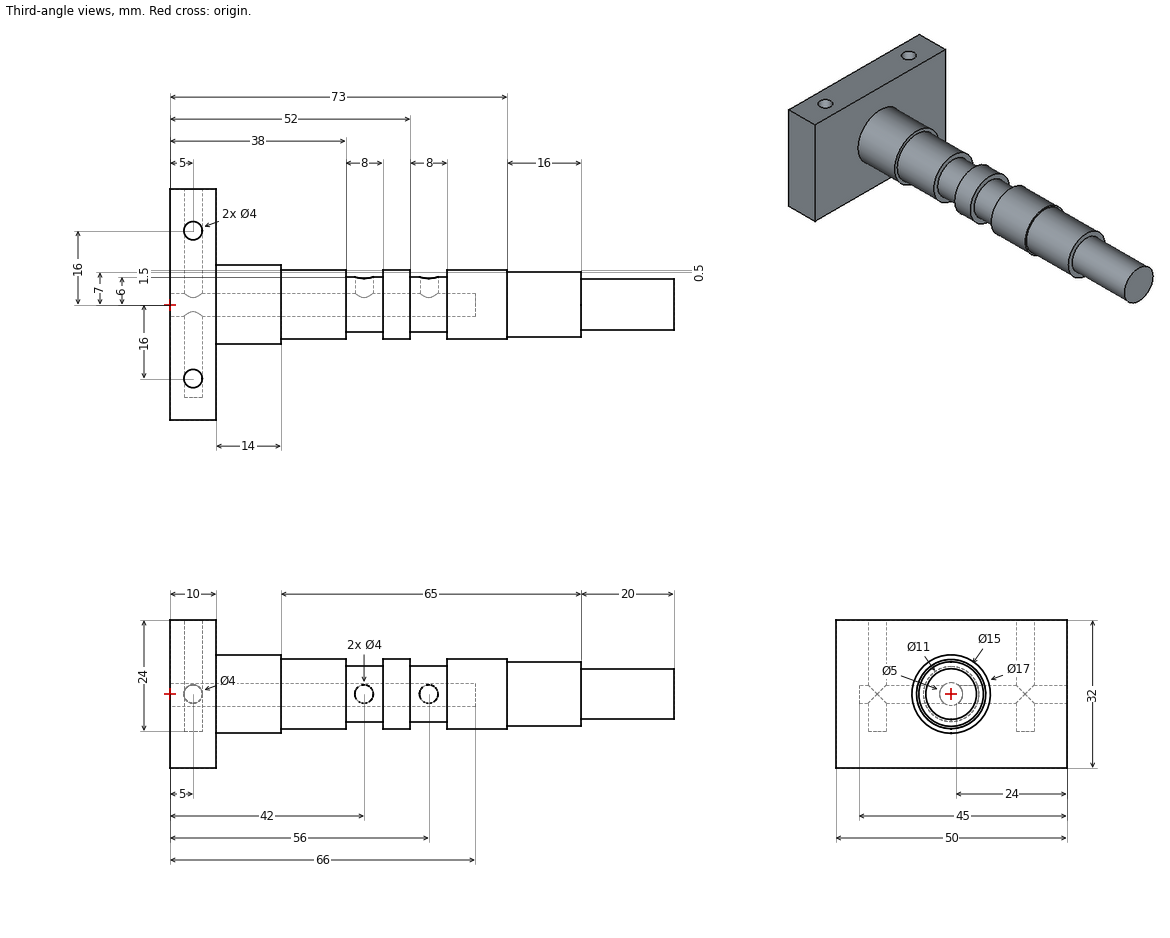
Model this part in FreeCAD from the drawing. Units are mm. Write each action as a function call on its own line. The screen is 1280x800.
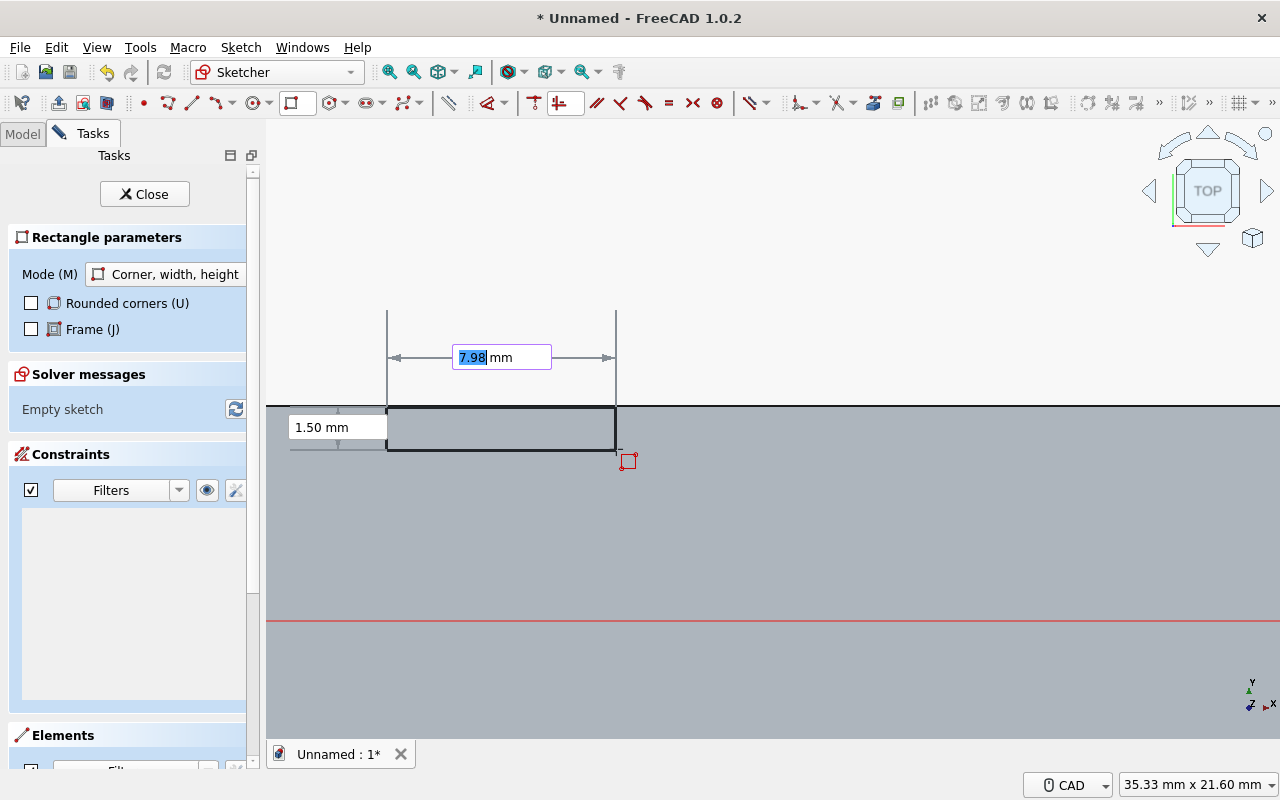
text(8)
key(Tab)
text(1.5)
key(Return)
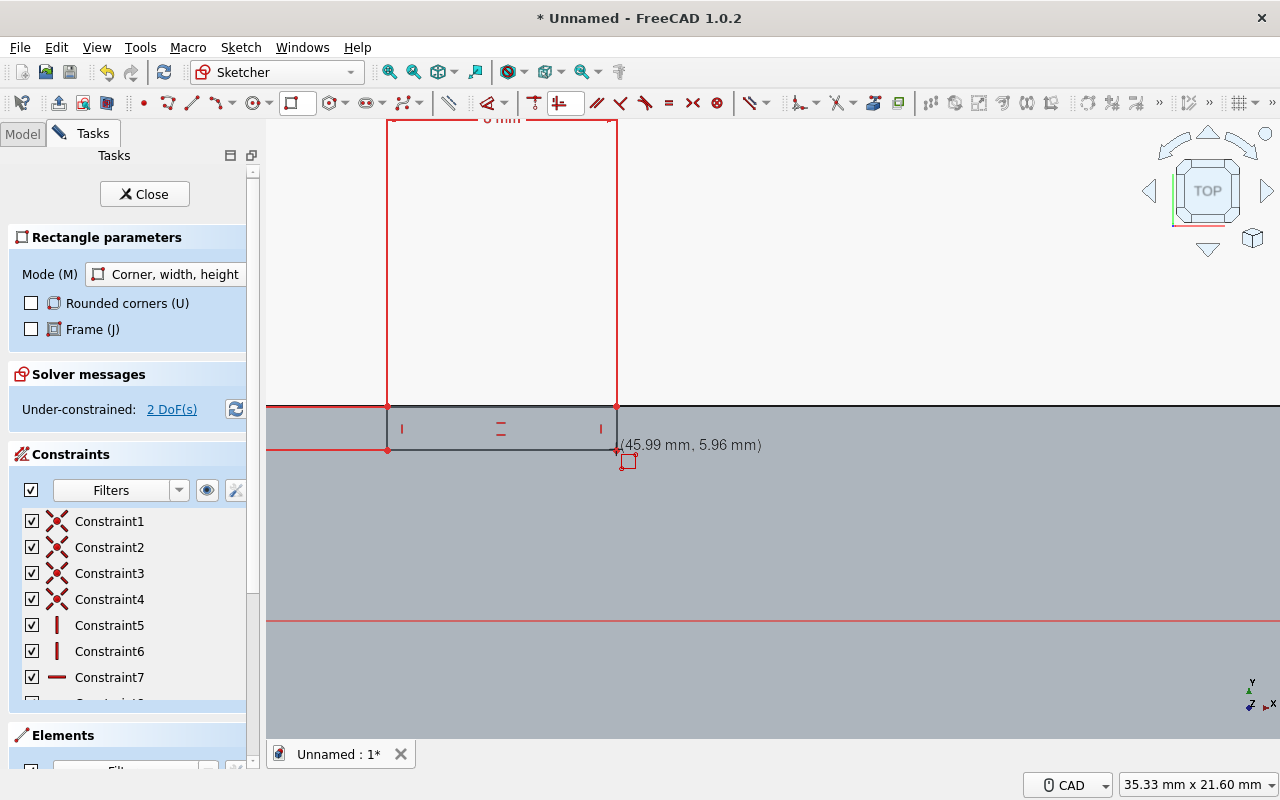
click(788, 406)
move(1018, 449)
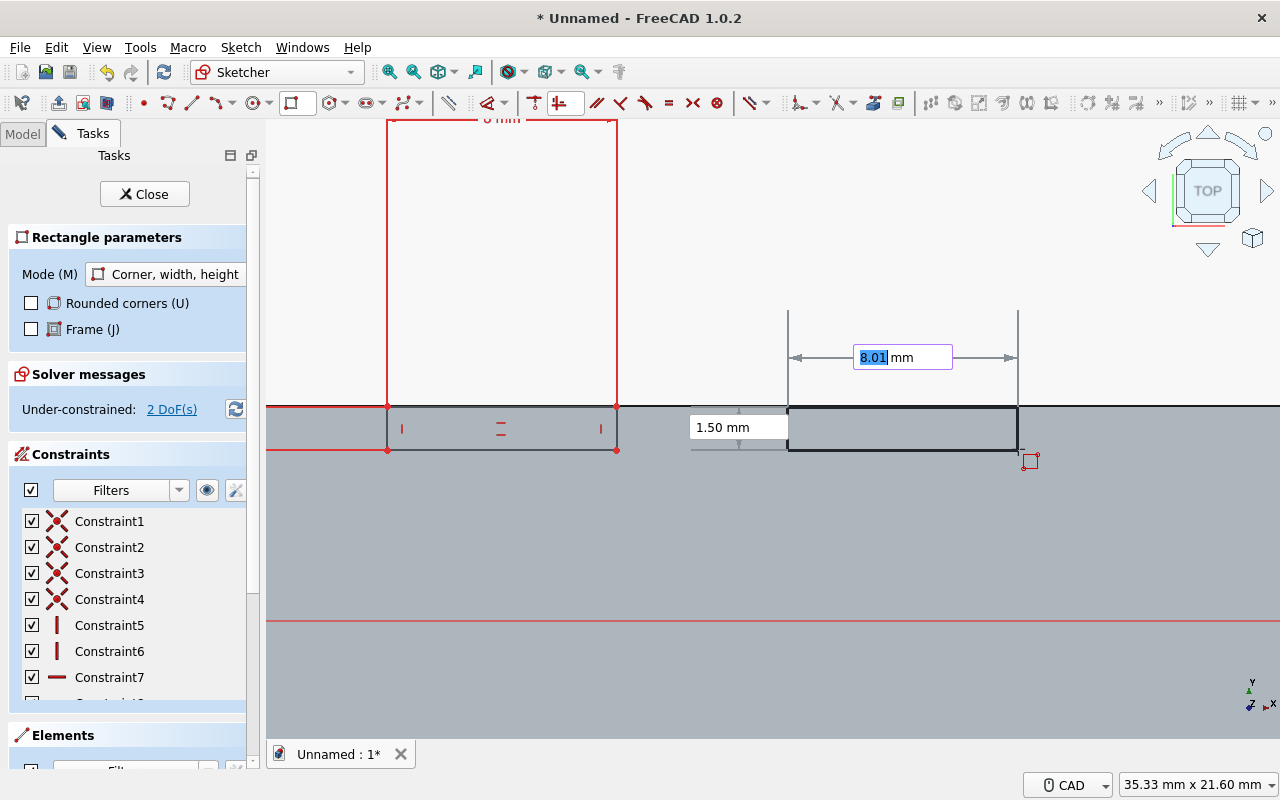
text(8)
key(Tab)
text(1.5)
key(Return)
key(Escape)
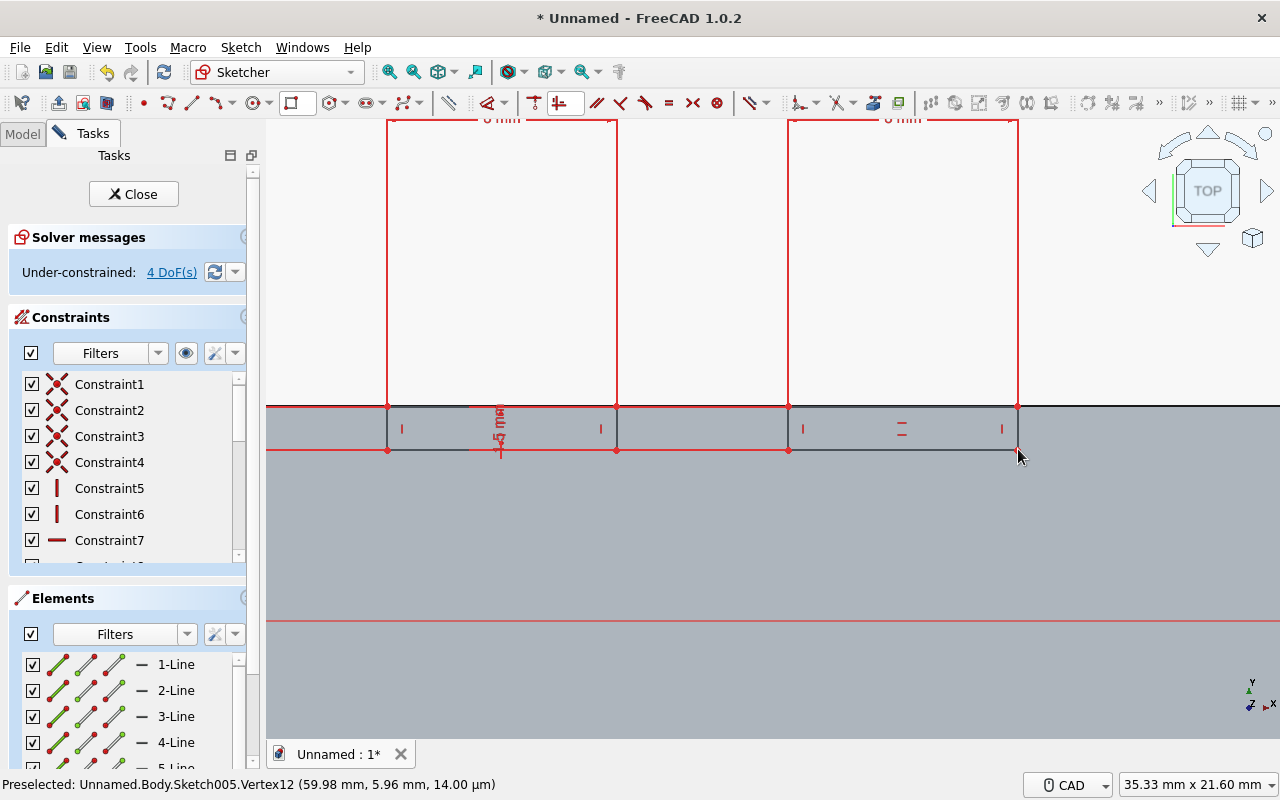
click(488, 104)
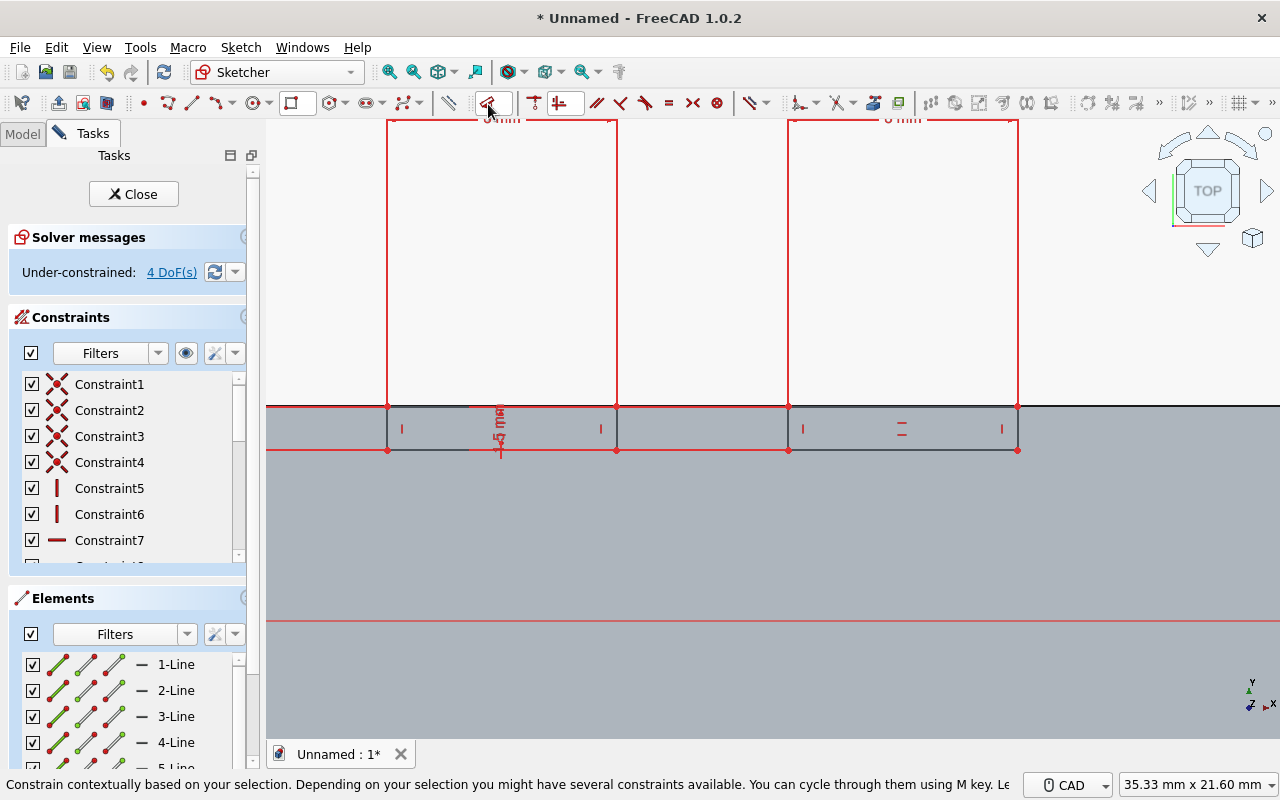
click(387, 450)
click(421, 536)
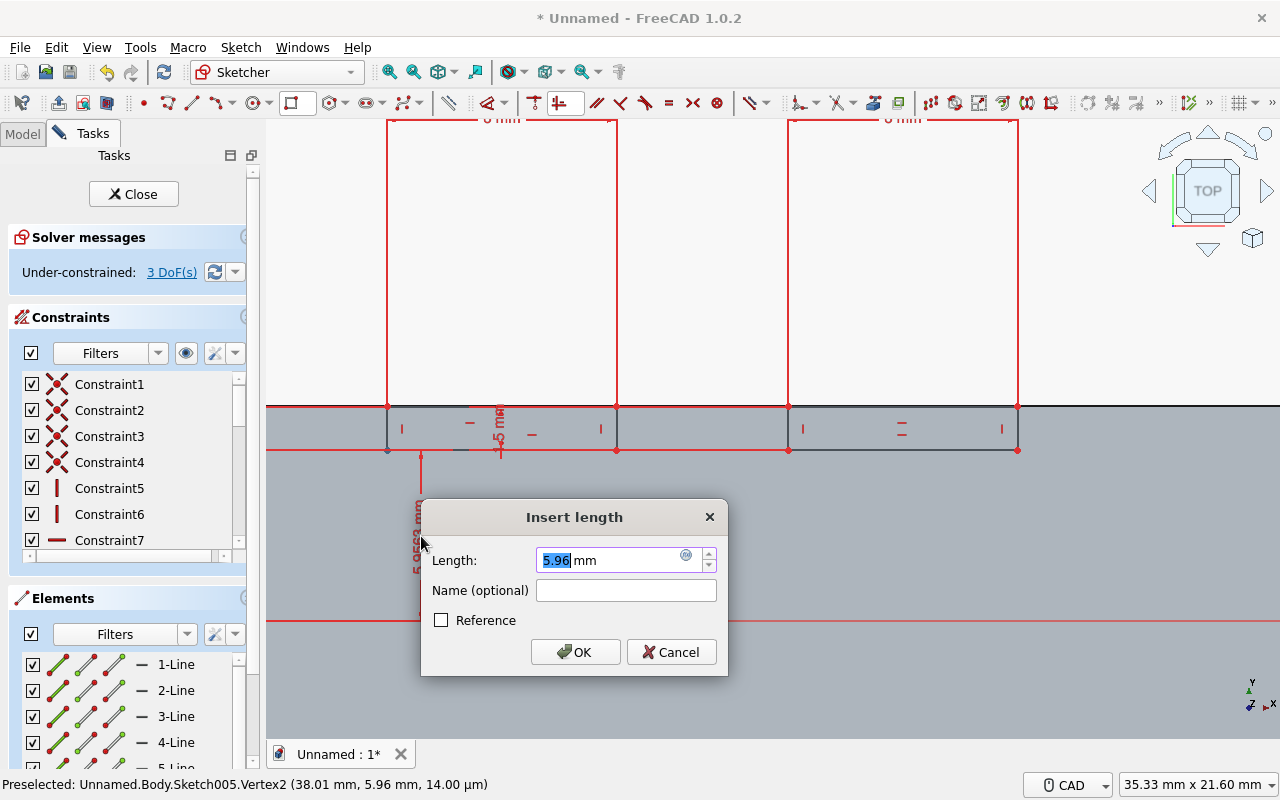
text(6)
key(Return)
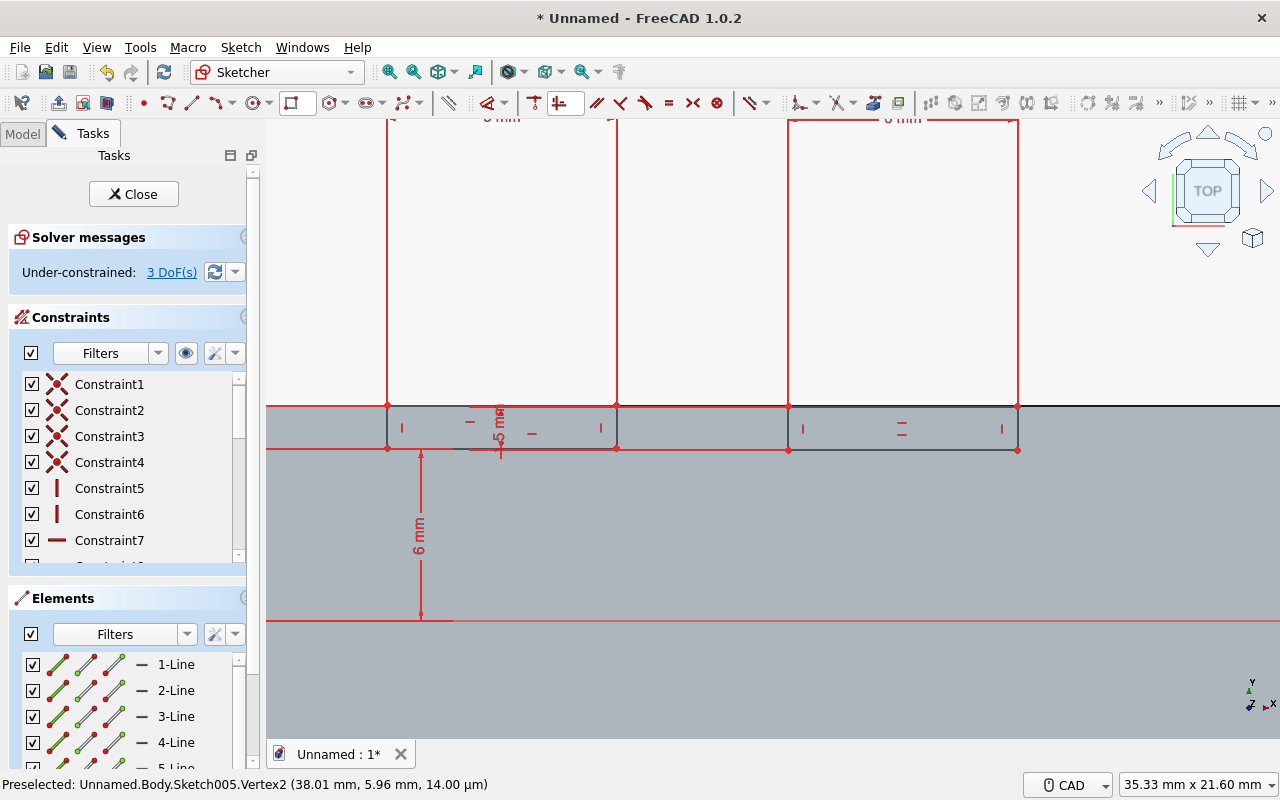
click(788, 450)
click(822, 536)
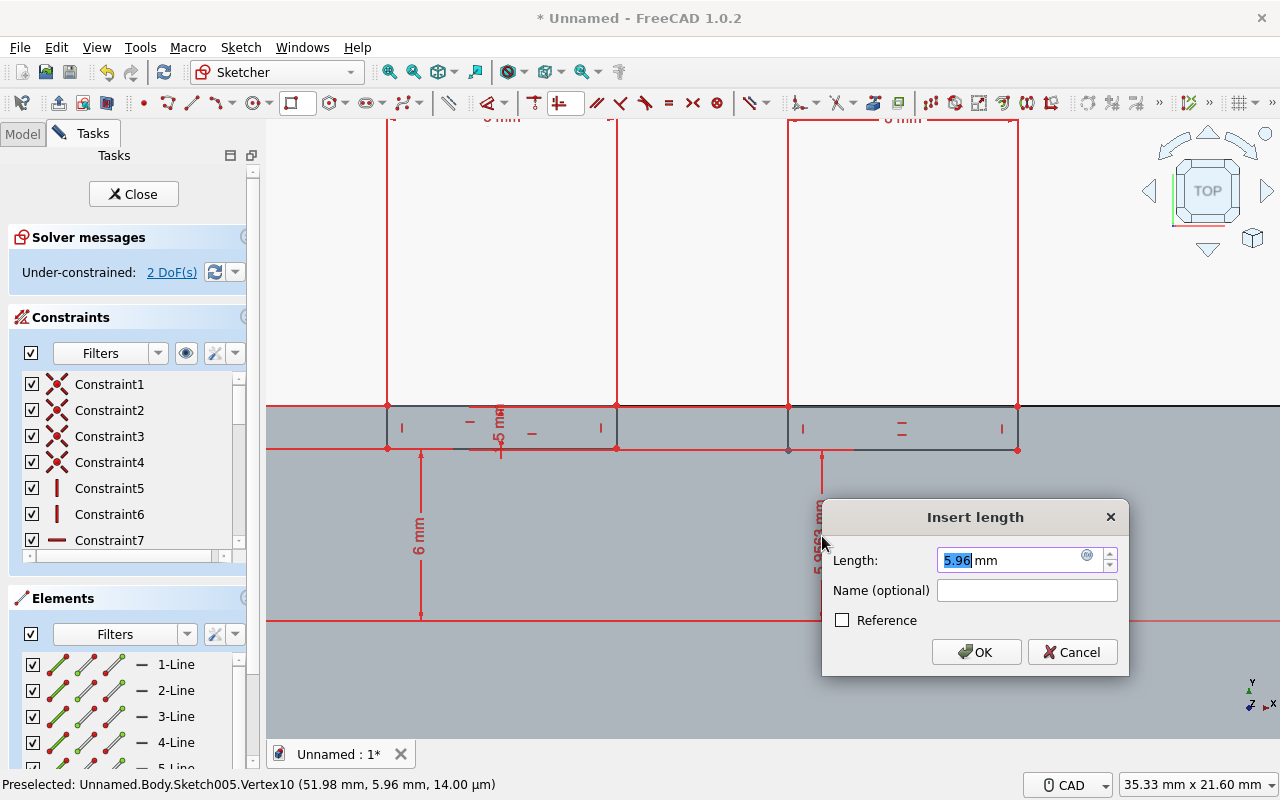
text(6)
key(Return)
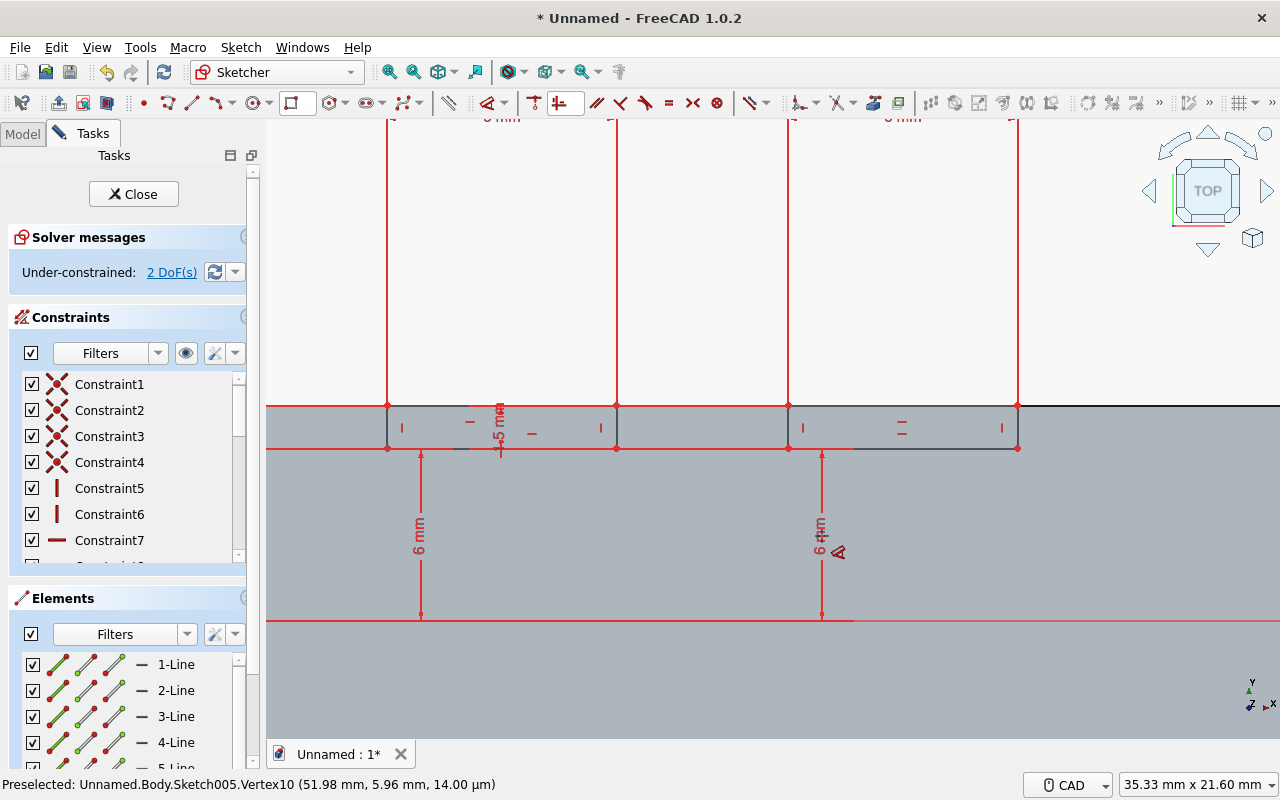
click(387, 406)
click(340, 655)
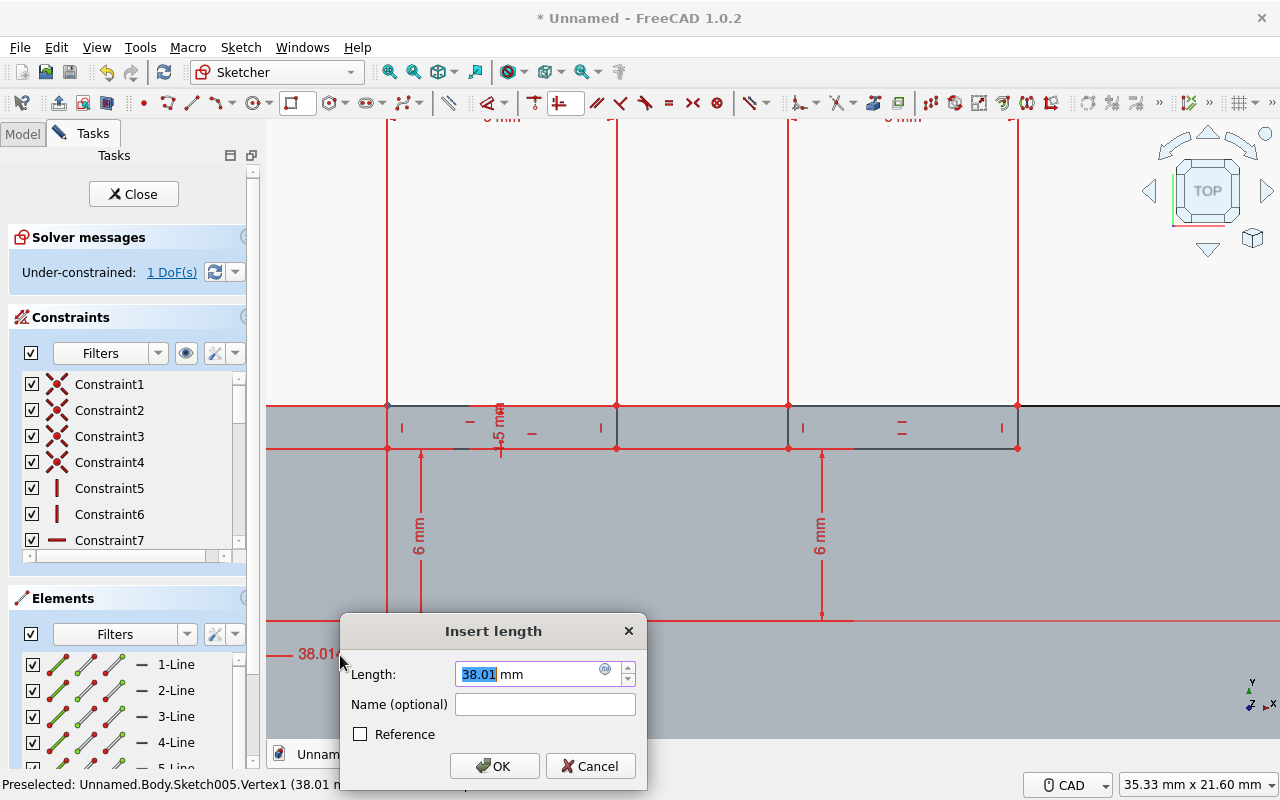
text(38)
key(Return)